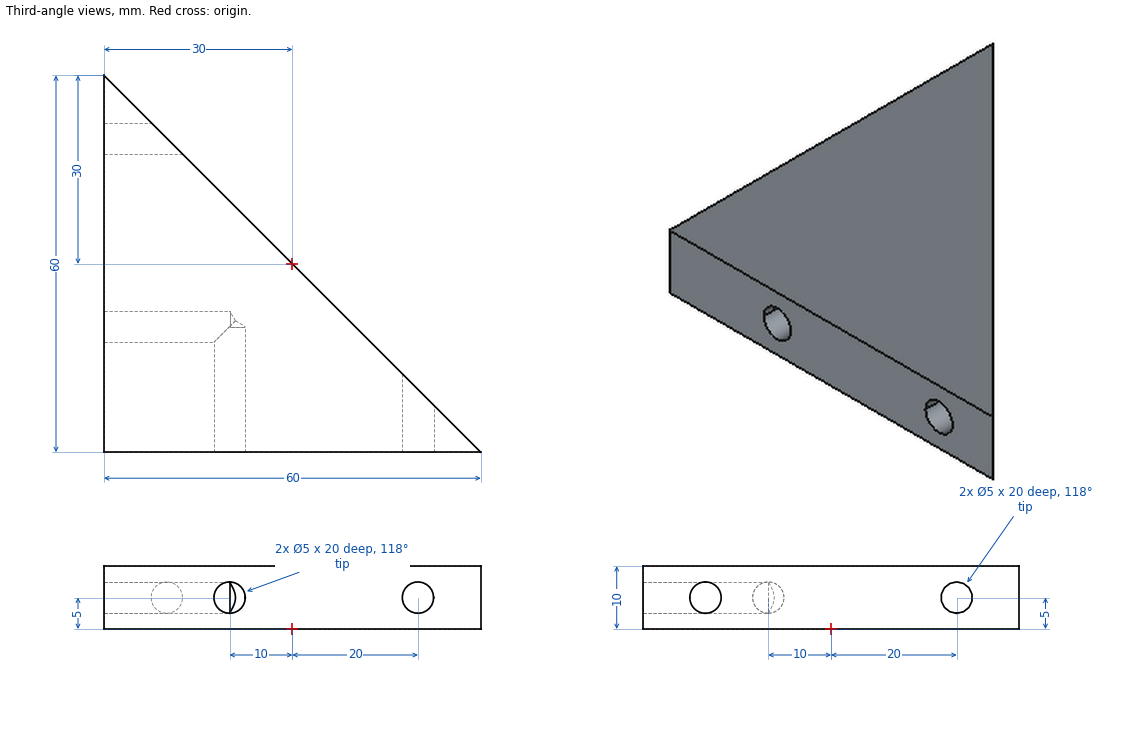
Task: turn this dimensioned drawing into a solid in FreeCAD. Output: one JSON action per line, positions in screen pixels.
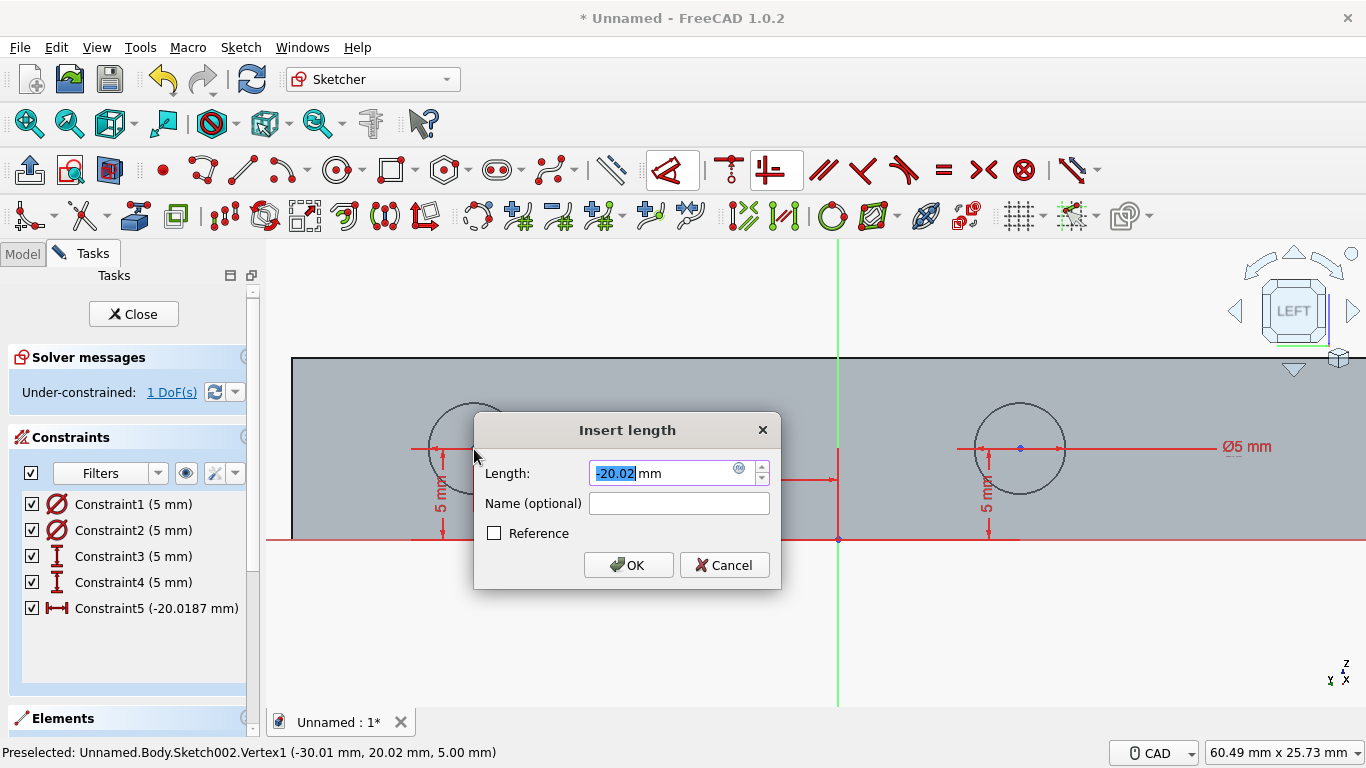
{"action": "type", "text": "-20"}
{"action": "key", "text": "Return"}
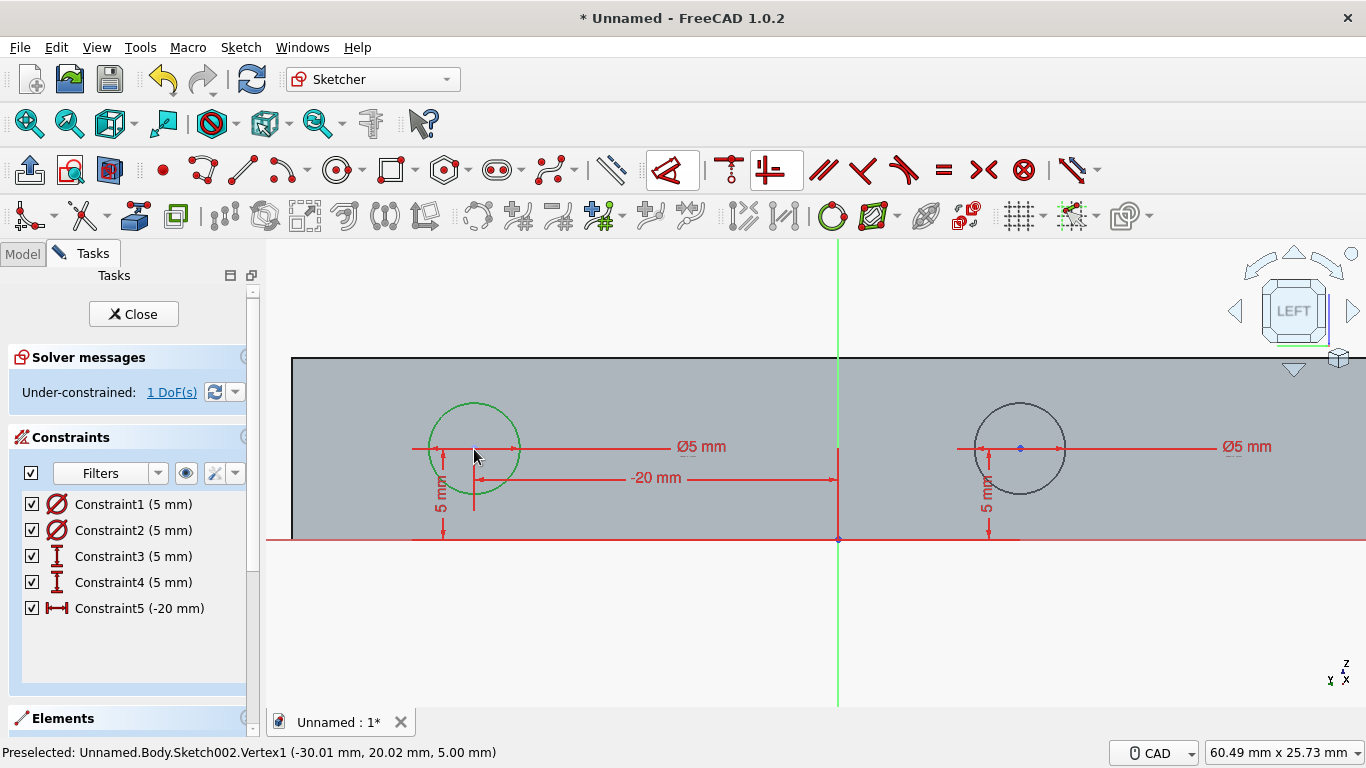
{"action": "left_click", "coordinate": [1020, 449]}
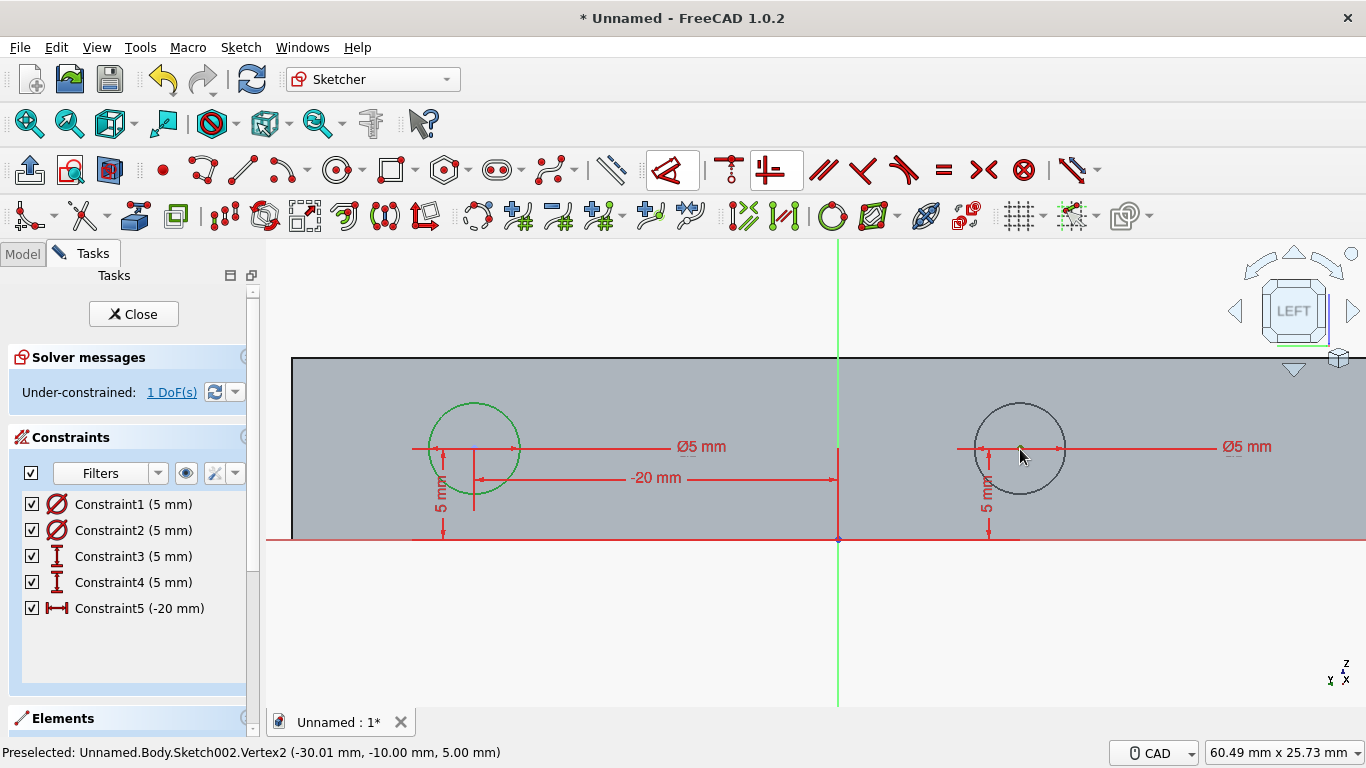
{"action": "key", "text": "l"}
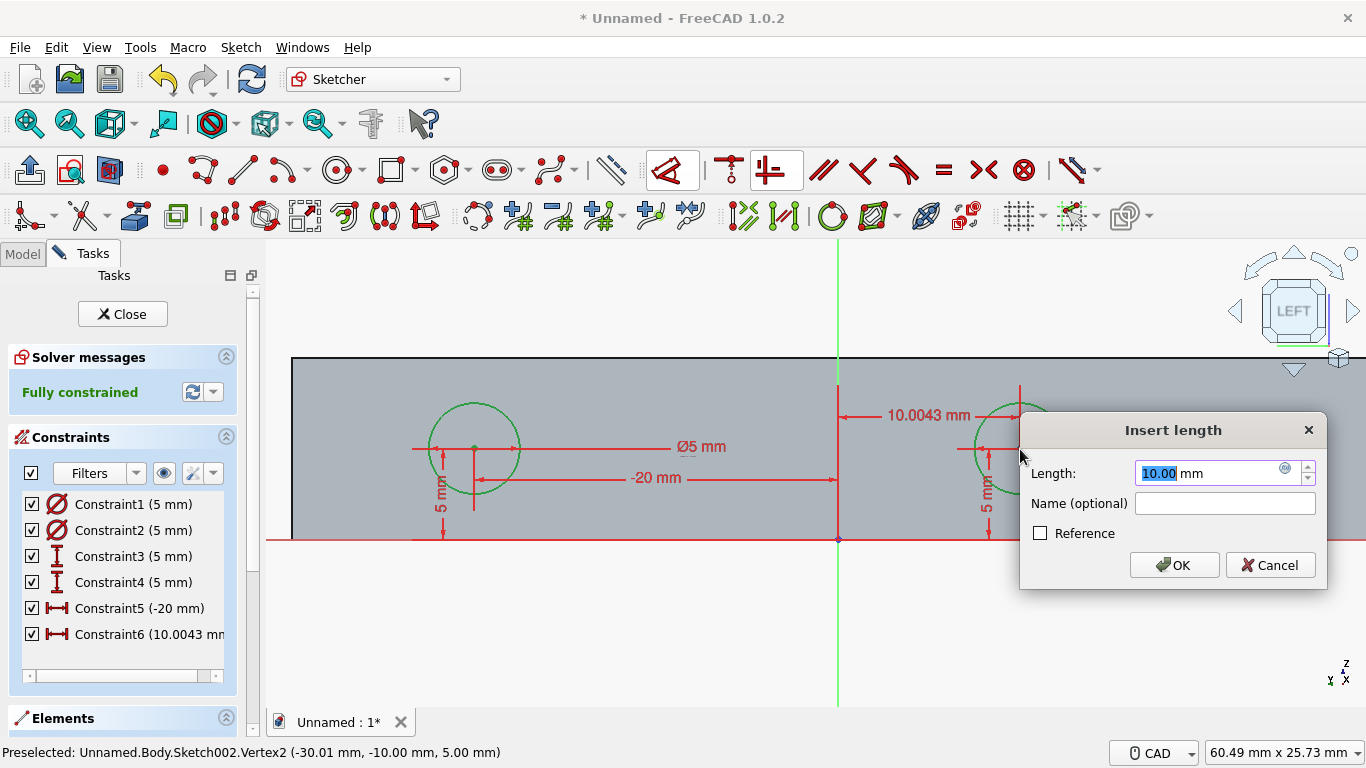
{"action": "type", "text": "10"}
{"action": "key", "text": "Return"}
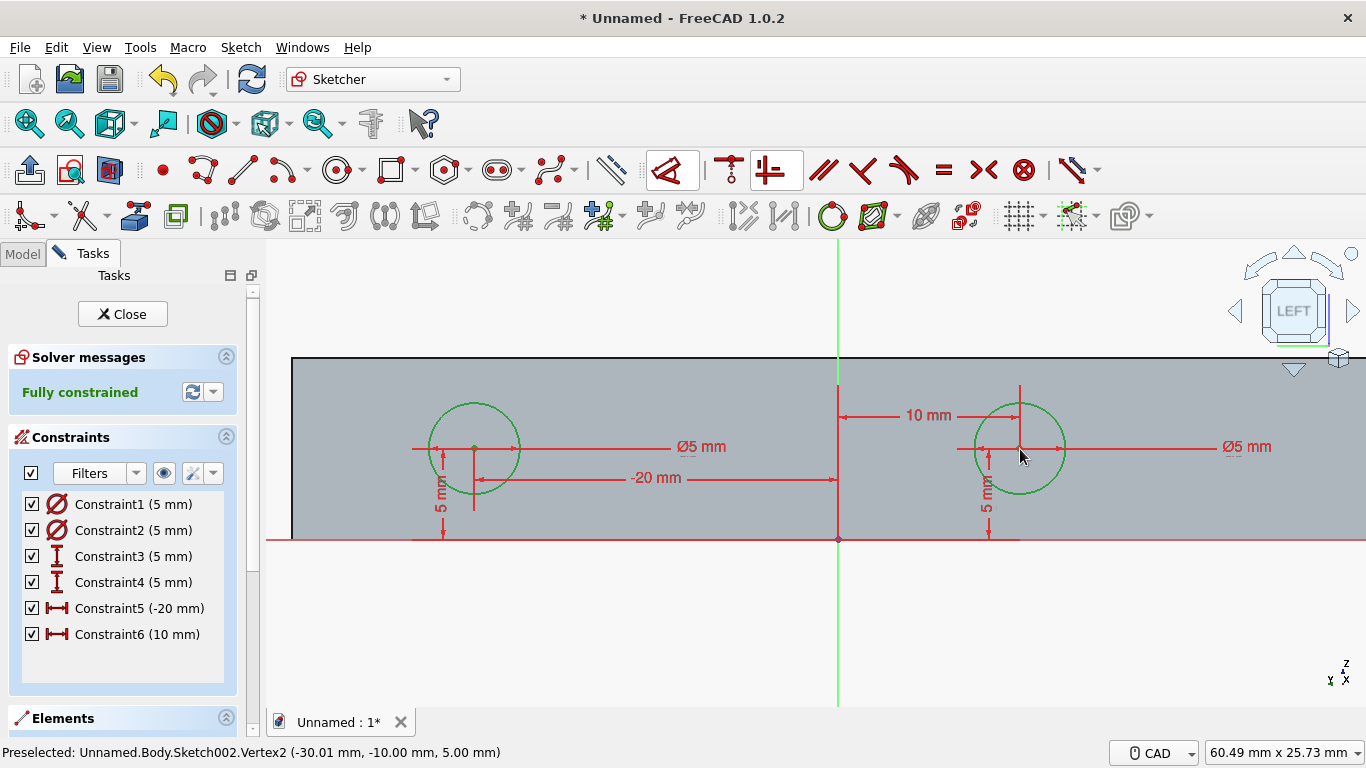
{"action": "left_click", "coordinate": [123, 314]}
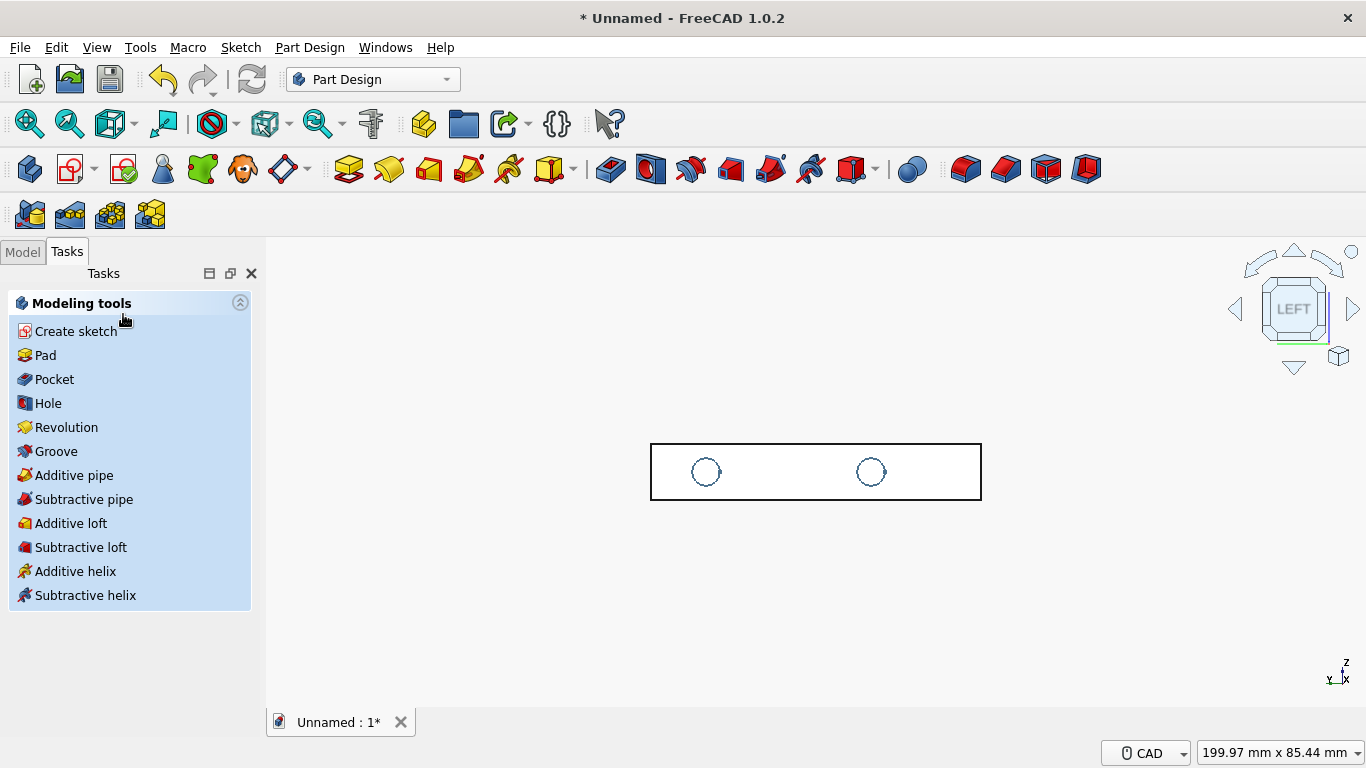
{"action": "left_click", "coordinate": [652, 170]}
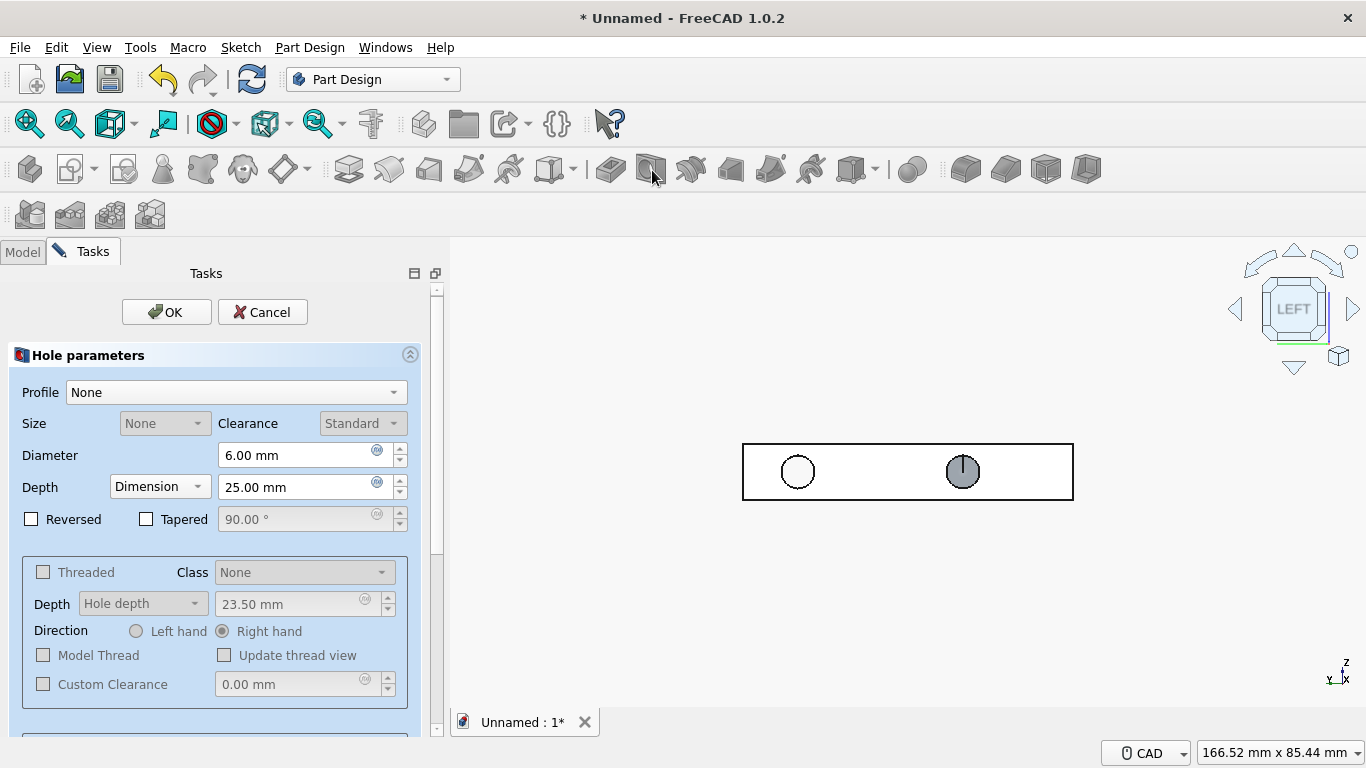
{"action": "triple_click", "coordinate": [305, 455]}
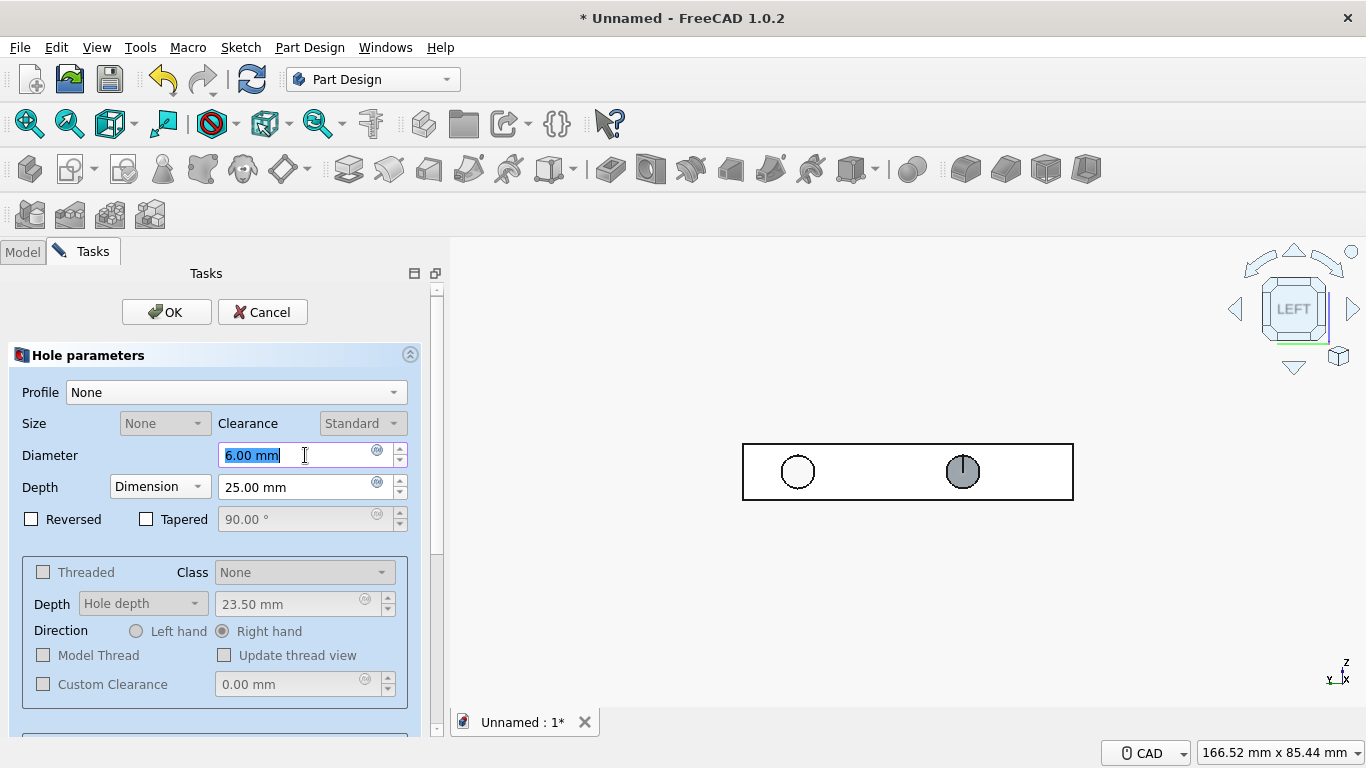
{"action": "type", "text": "5"}
{"action": "key", "text": "Tab"}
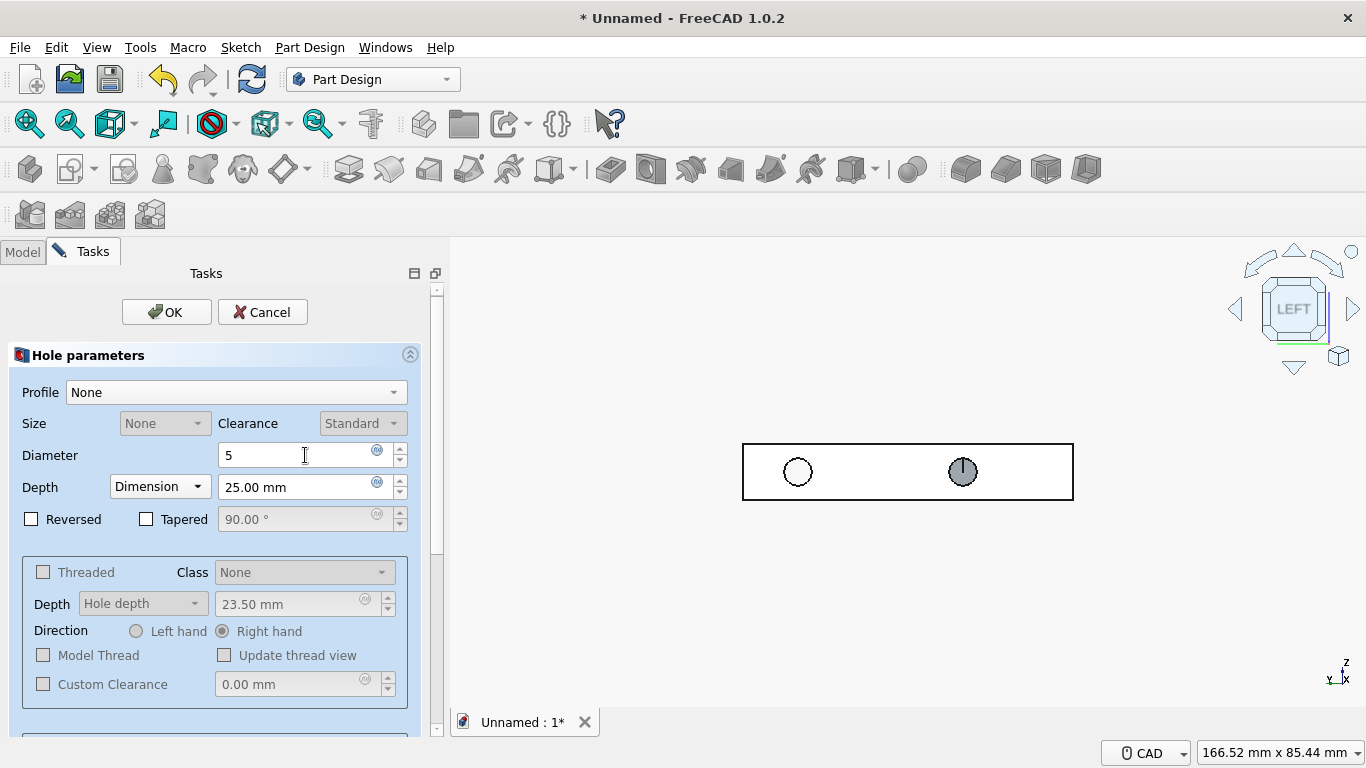
{"action": "triple_click", "coordinate": [305, 487]}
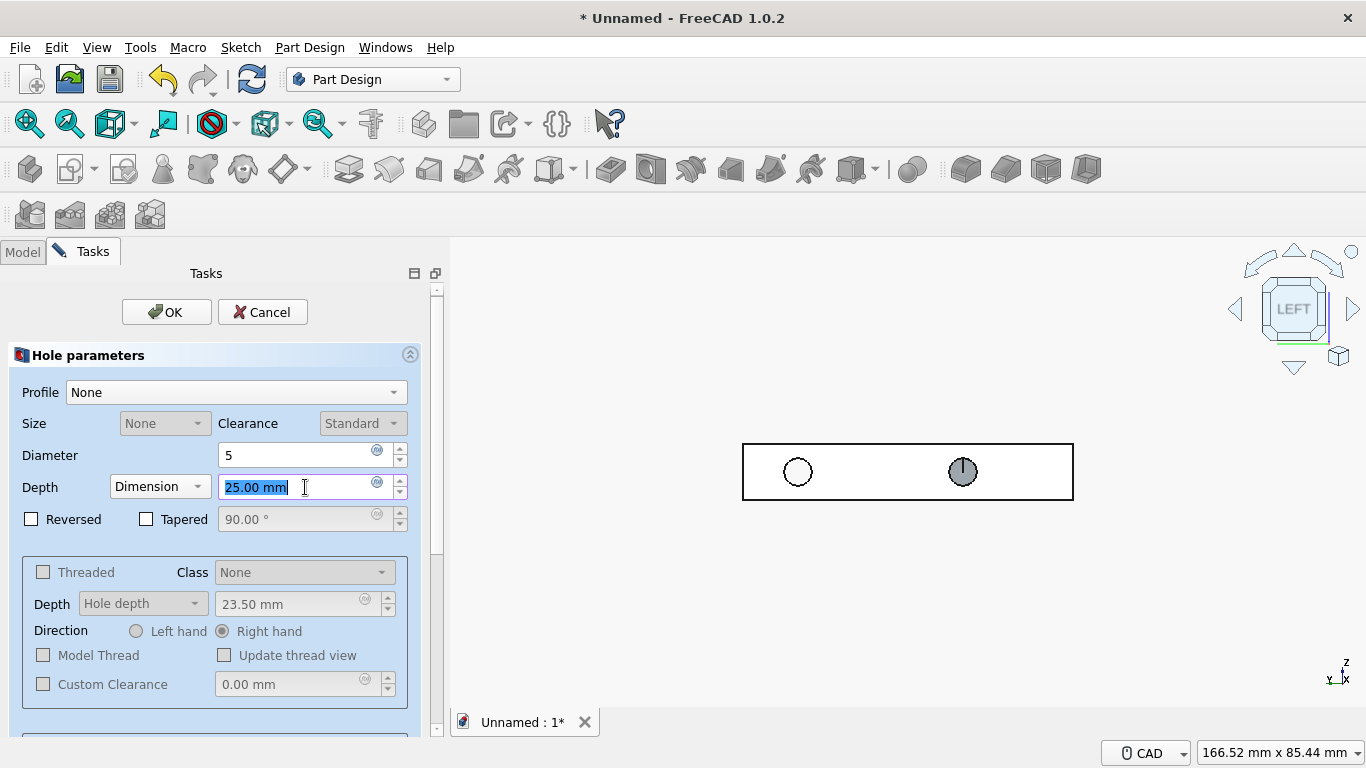
{"action": "type", "text": "20"}
{"action": "key", "text": "Tab"}